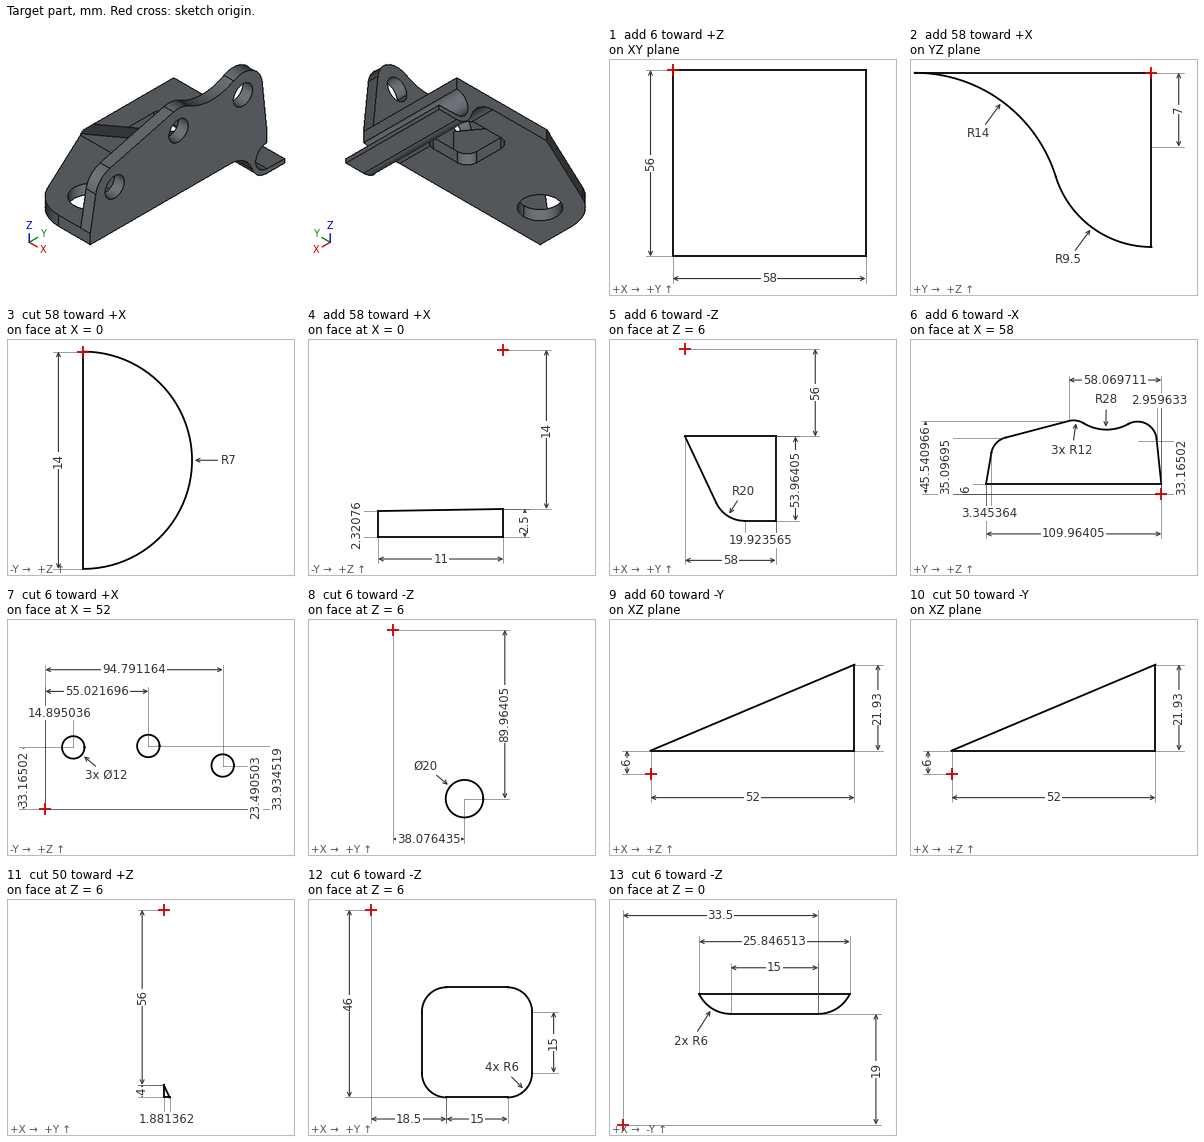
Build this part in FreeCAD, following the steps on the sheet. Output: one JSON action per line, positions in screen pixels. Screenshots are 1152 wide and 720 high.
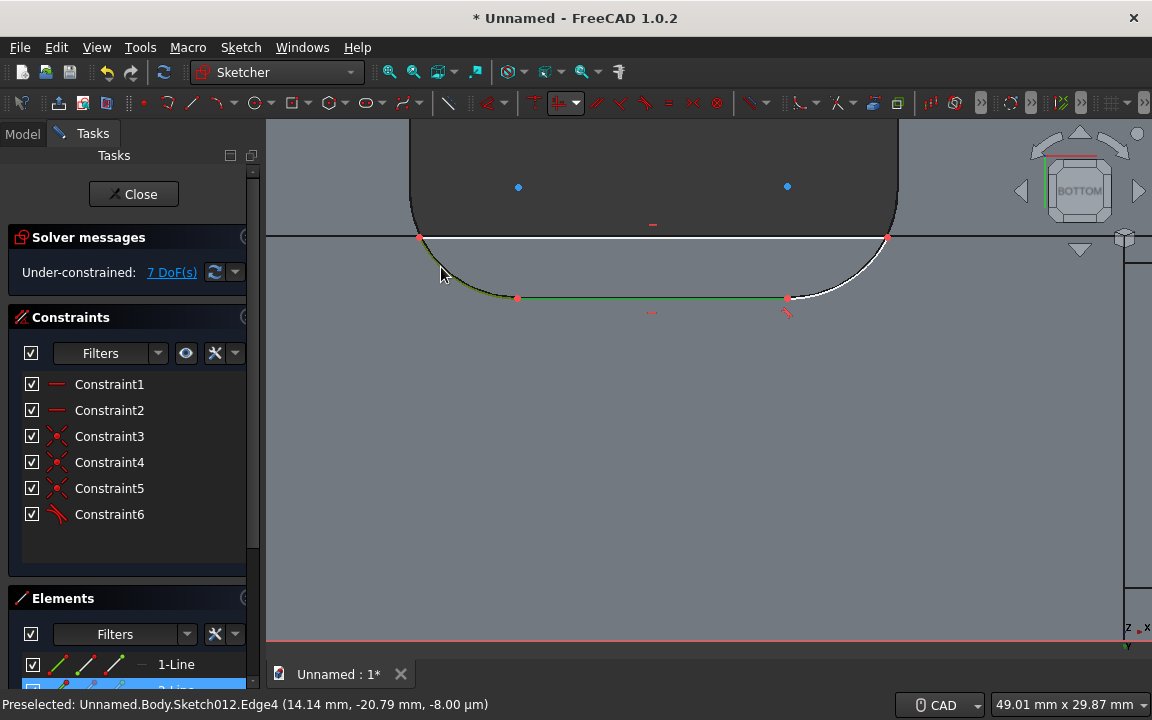
{"action": "key", "text": "t"}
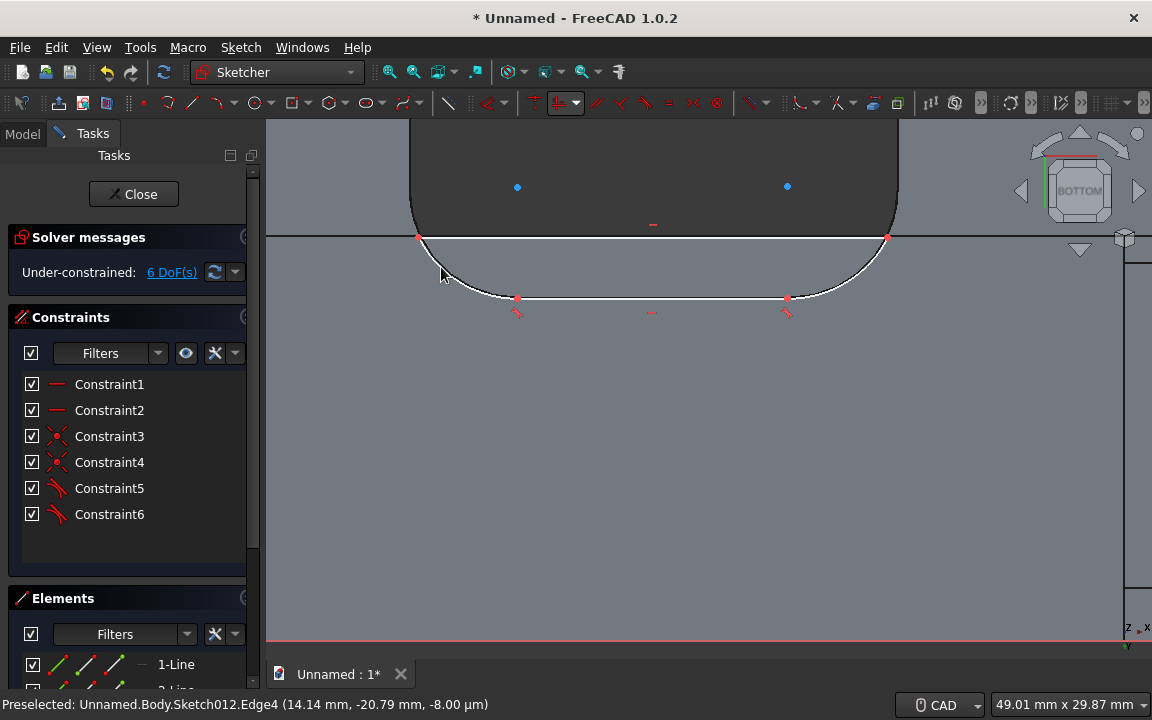
{"action": "left_click", "coordinate": [824, 293]}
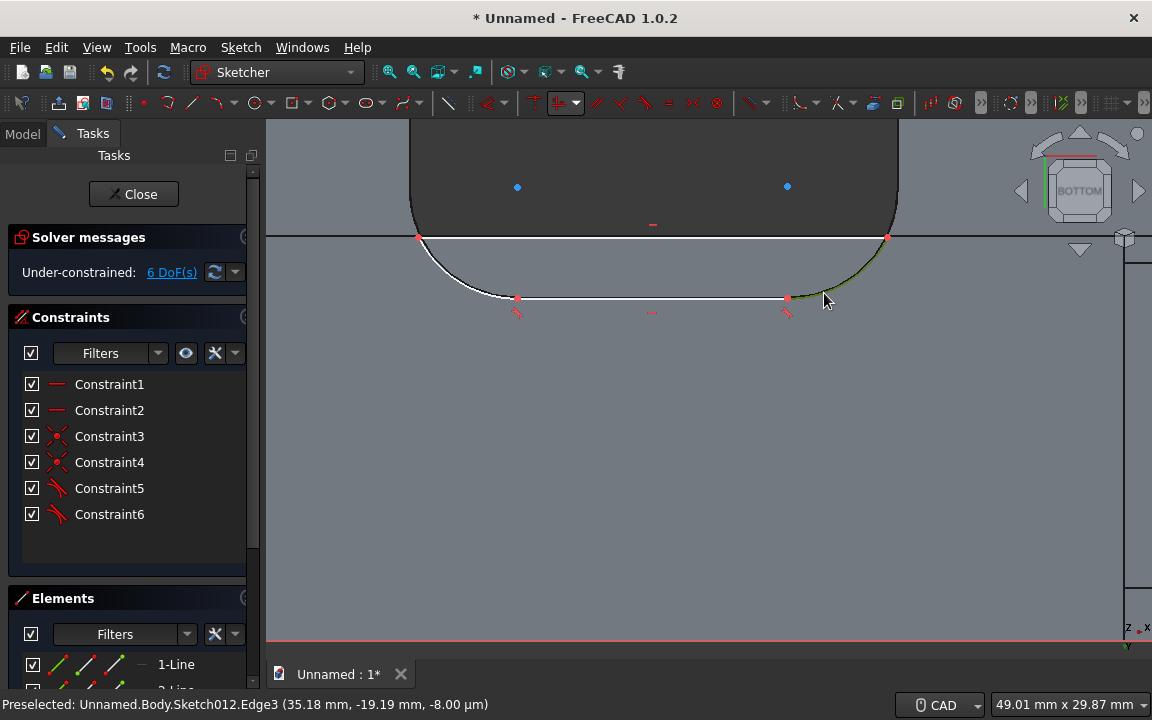
{"action": "left_click", "coordinate": [440, 267]}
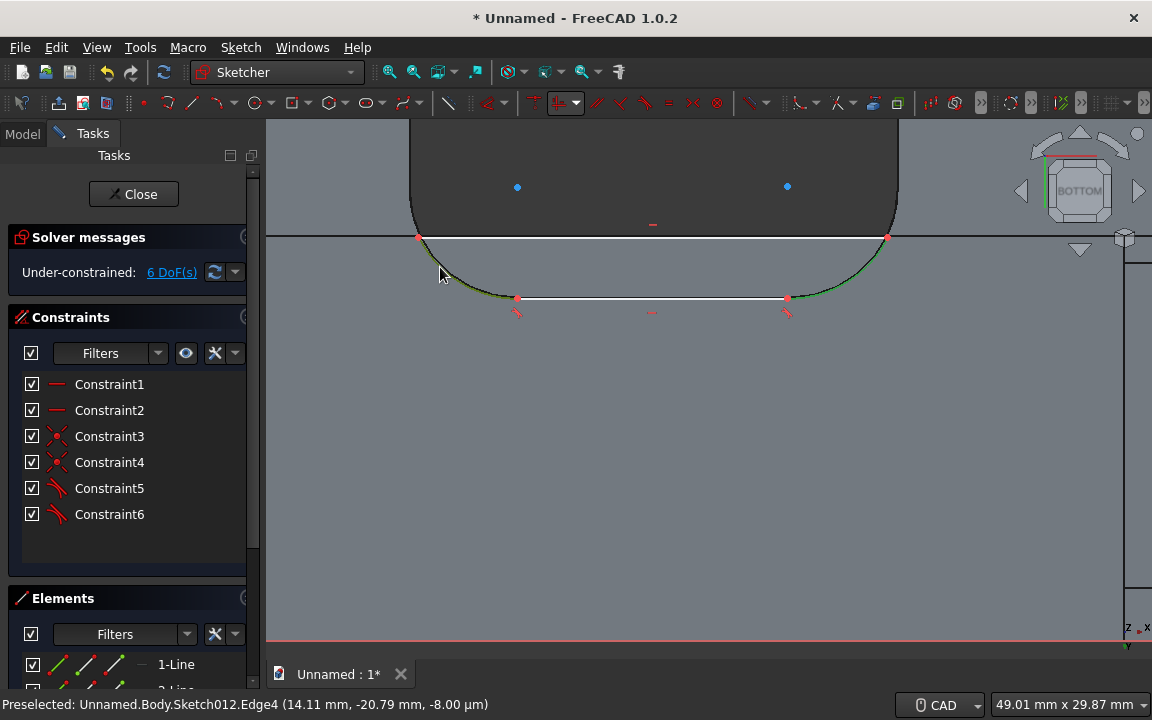
{"action": "left_click", "coordinate": [670, 104]}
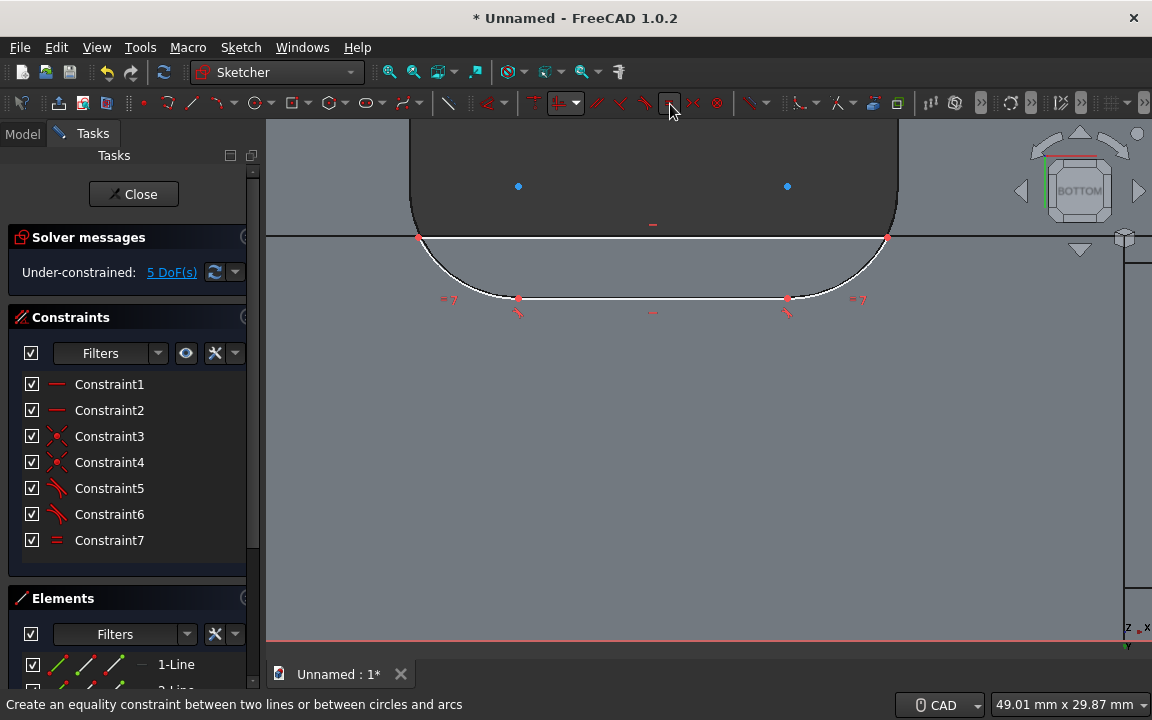
{"action": "left_click", "coordinate": [488, 104]}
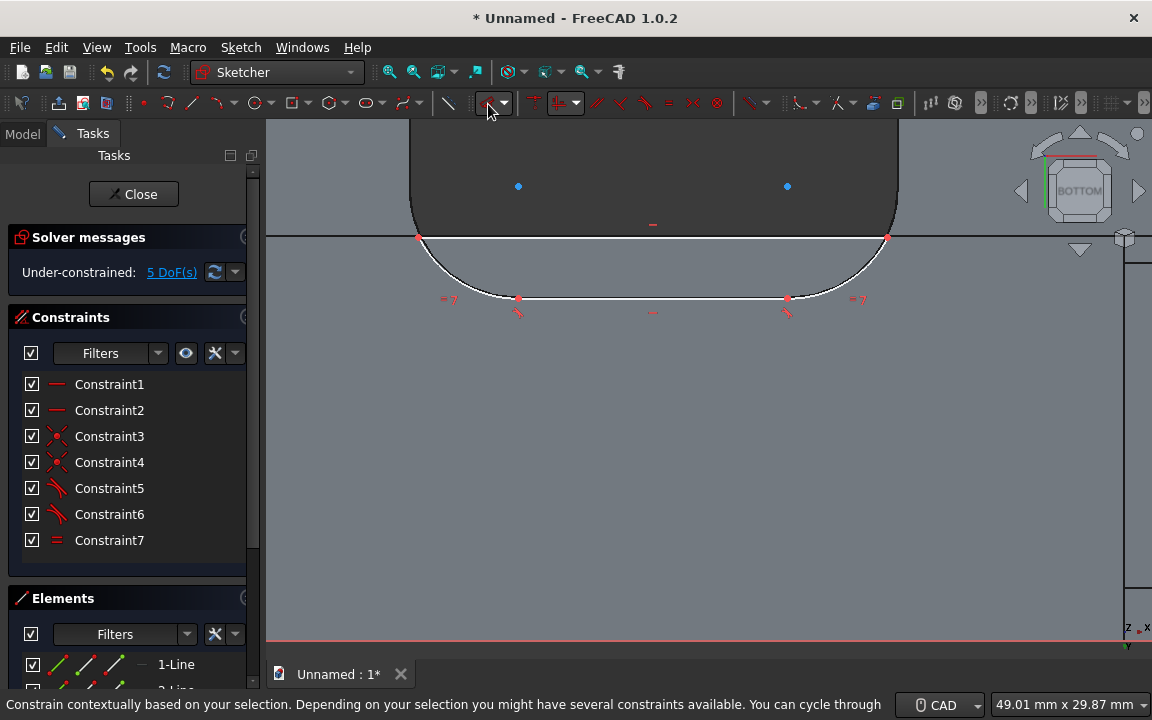
{"action": "left_click", "coordinate": [824, 293]}
{"action": "left_click", "coordinate": [834, 323]}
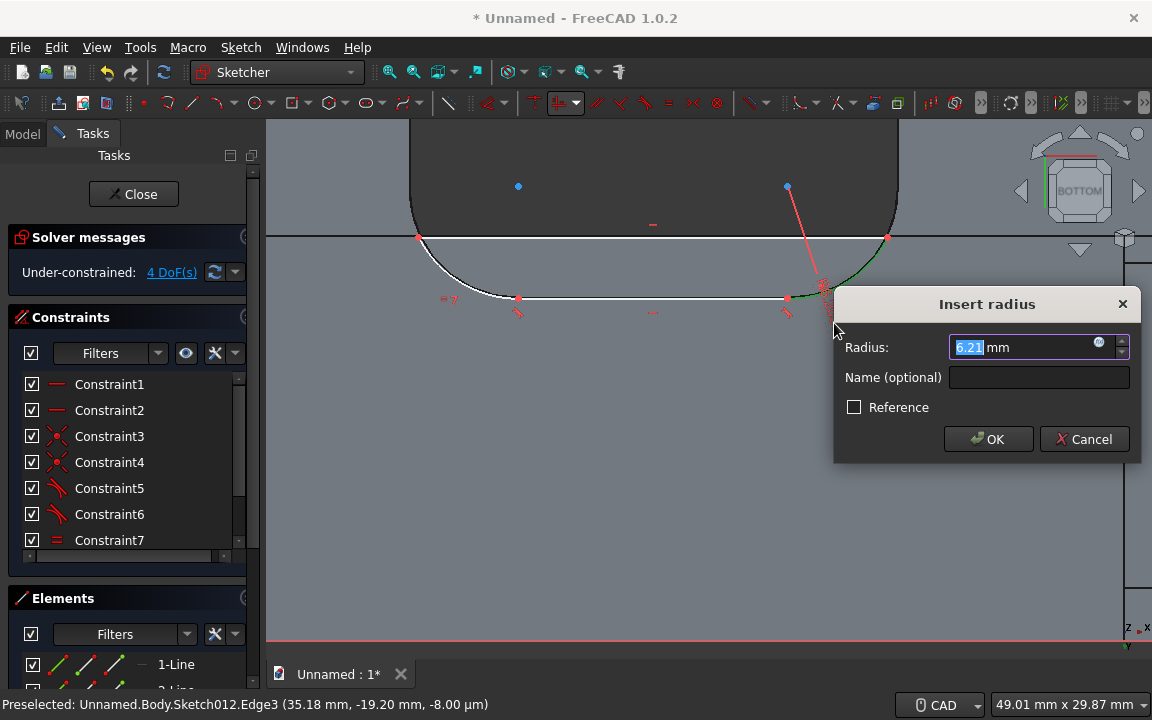
{"action": "type", "text": "6"}
{"action": "key", "text": "Return"}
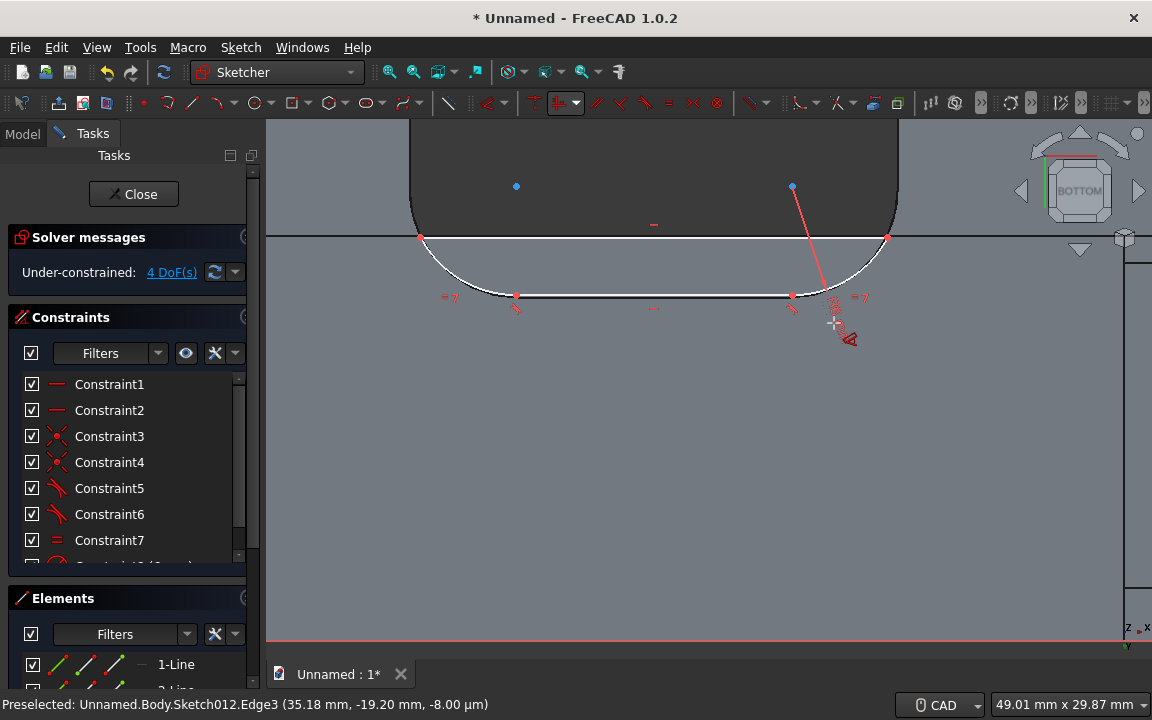
{"action": "left_click", "coordinate": [709, 295]}
{"action": "left_click", "coordinate": [654, 261]}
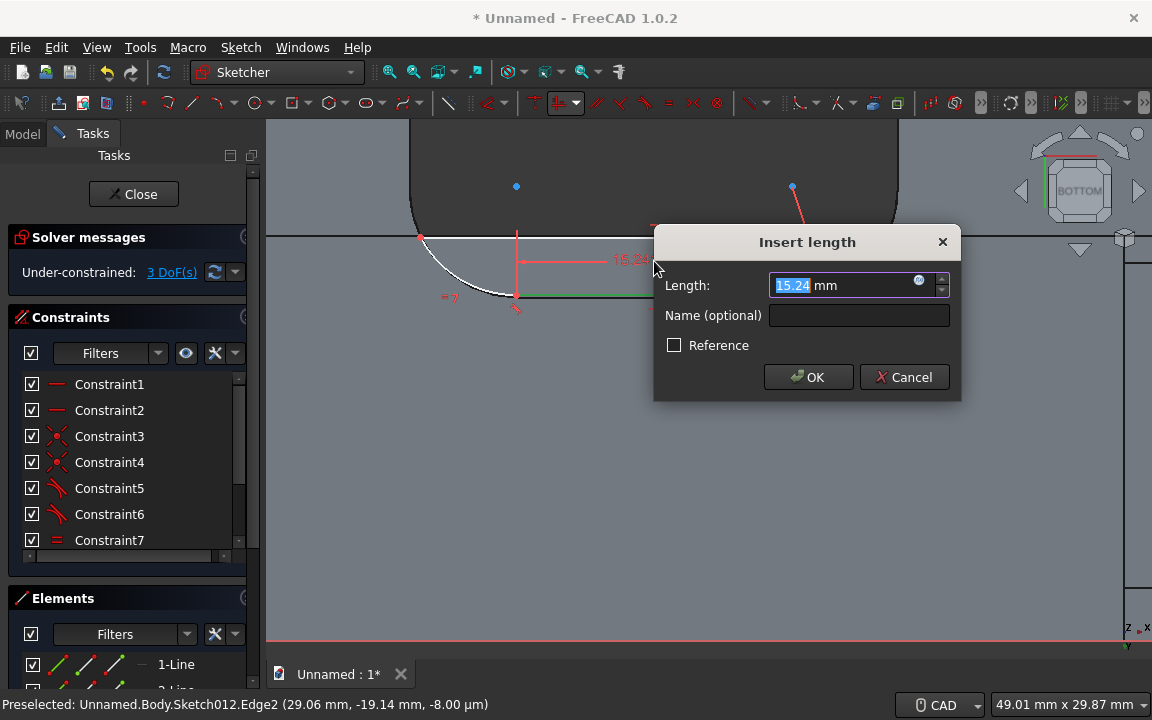
{"action": "type", "text": "15"}
{"action": "key", "text": "Return"}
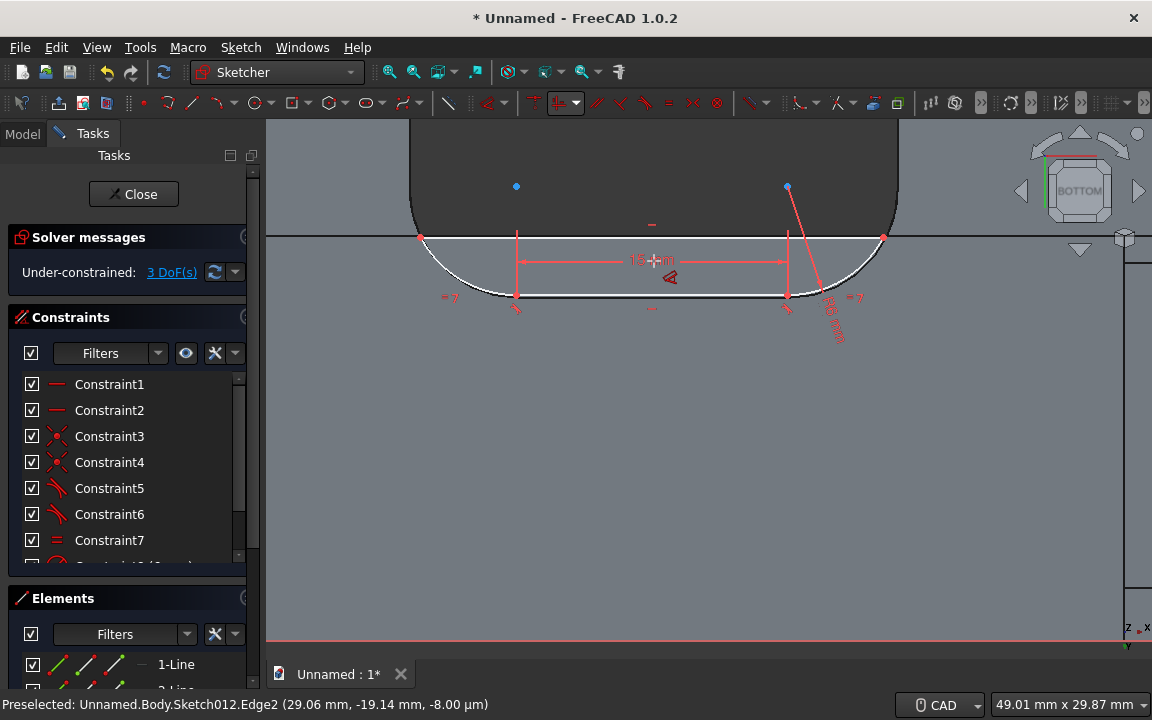
{"action": "left_click", "coordinate": [788, 295]}
{"action": "left_click", "coordinate": [822, 463]}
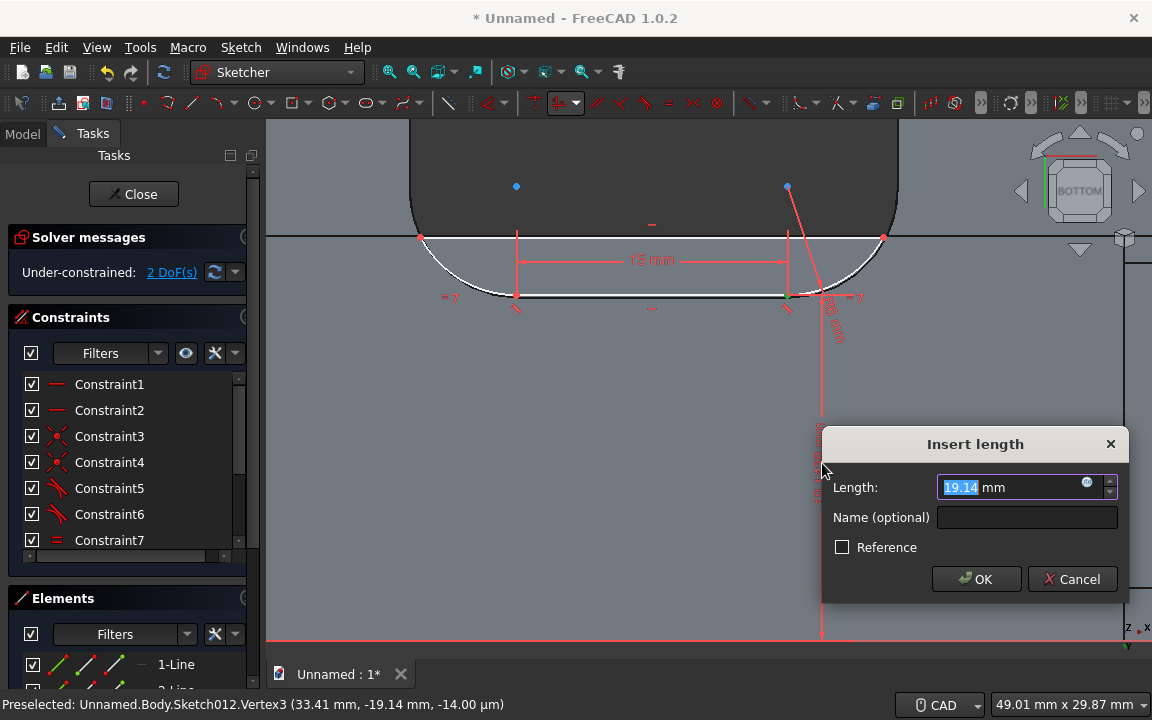
{"action": "type", "text": "19"}
{"action": "key", "text": "Return"}